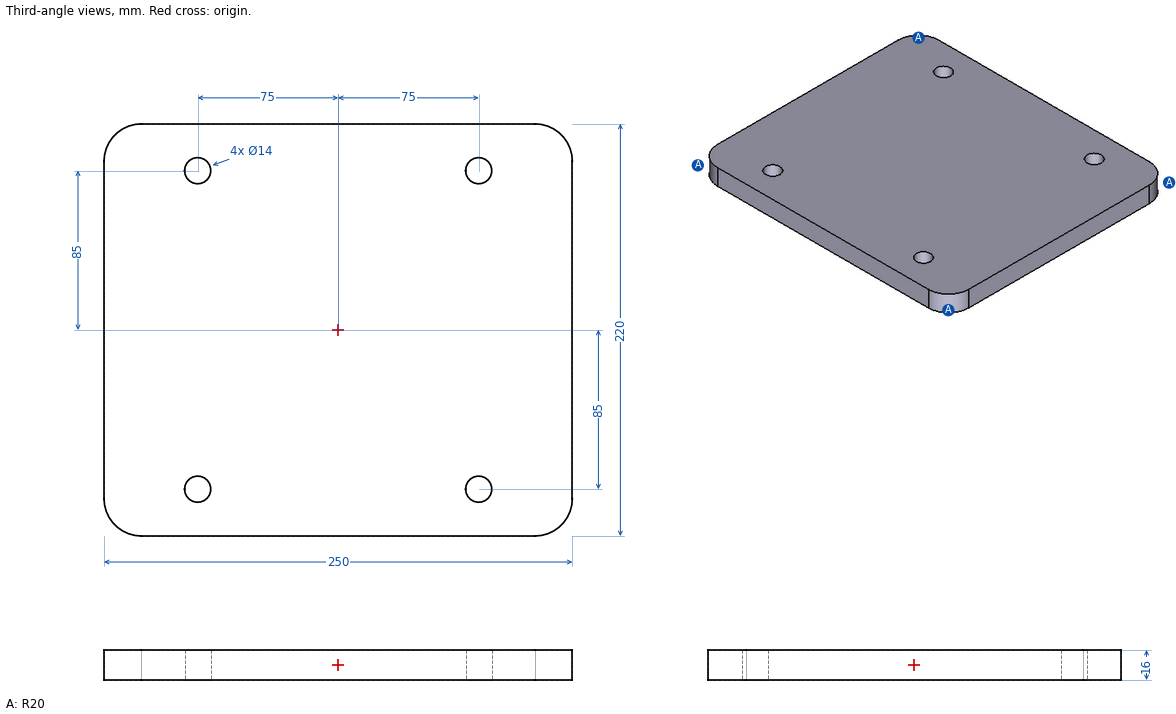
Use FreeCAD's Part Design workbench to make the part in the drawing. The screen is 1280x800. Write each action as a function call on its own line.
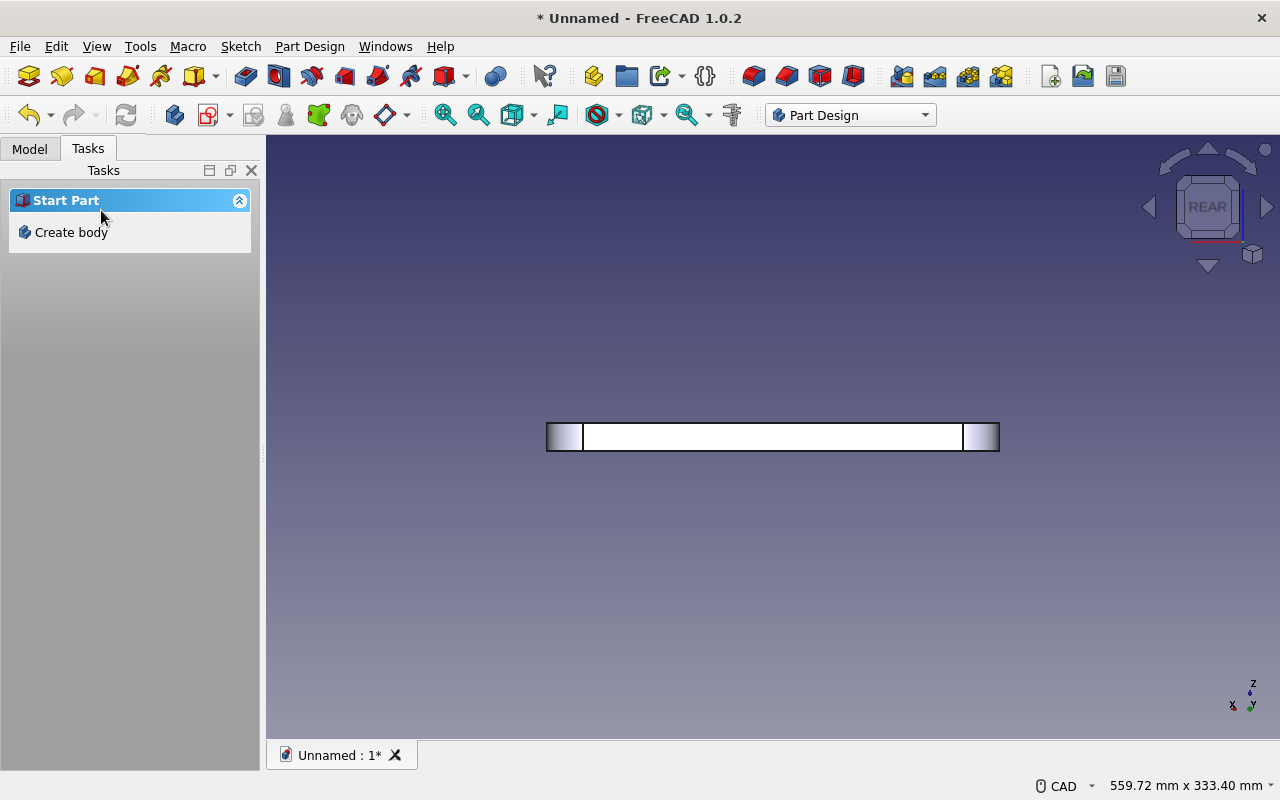
key(0)